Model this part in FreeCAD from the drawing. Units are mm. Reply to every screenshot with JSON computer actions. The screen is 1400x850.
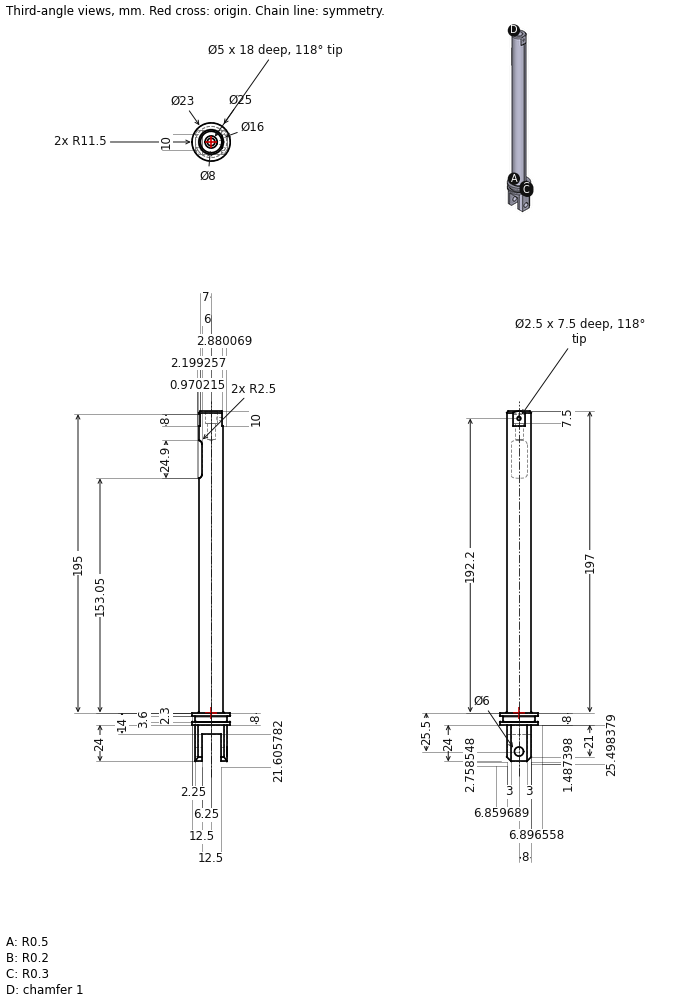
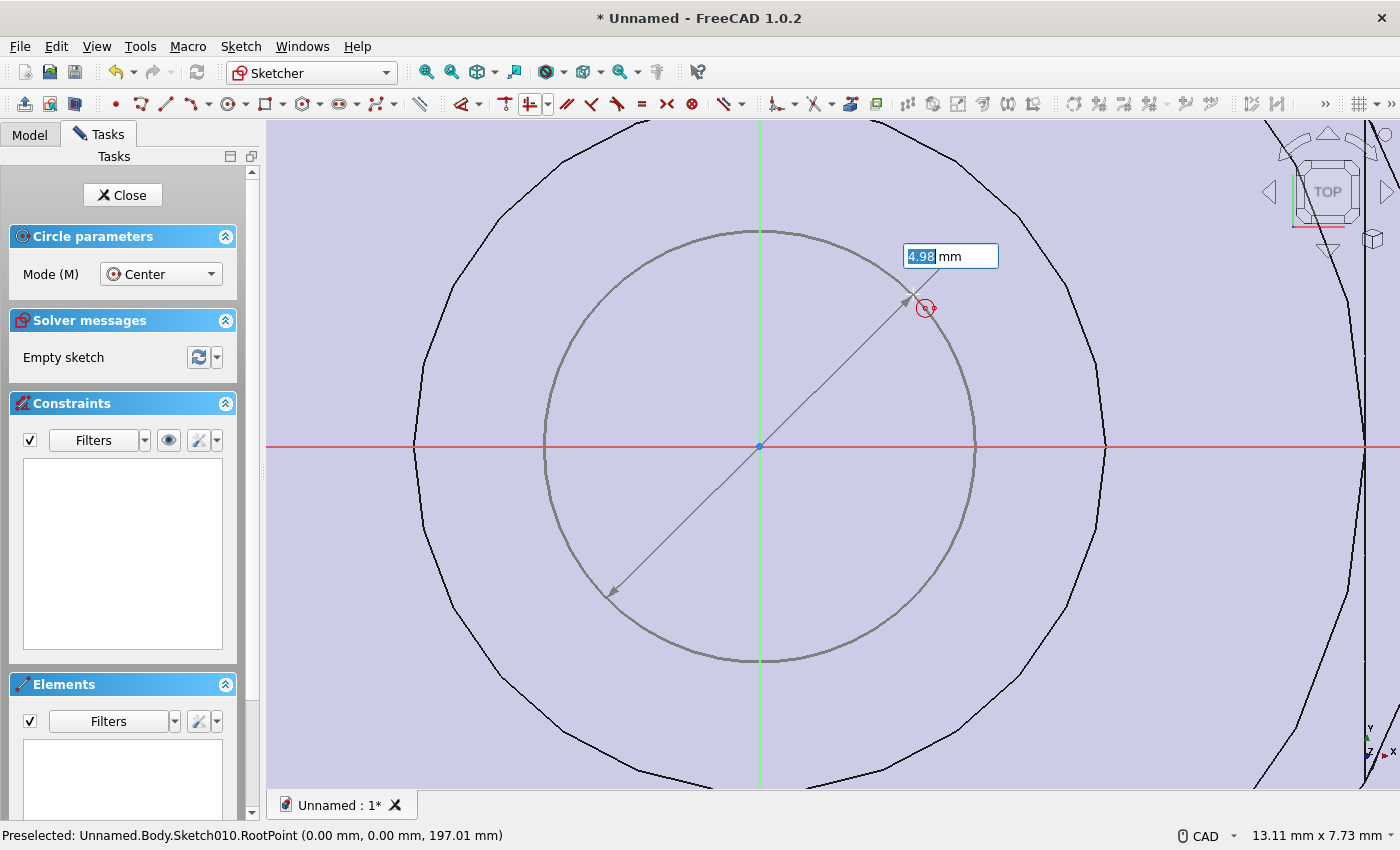
{"action": "type", "text": "5"}
{"action": "key", "text": "Return"}
{"action": "key", "text": "Escape"}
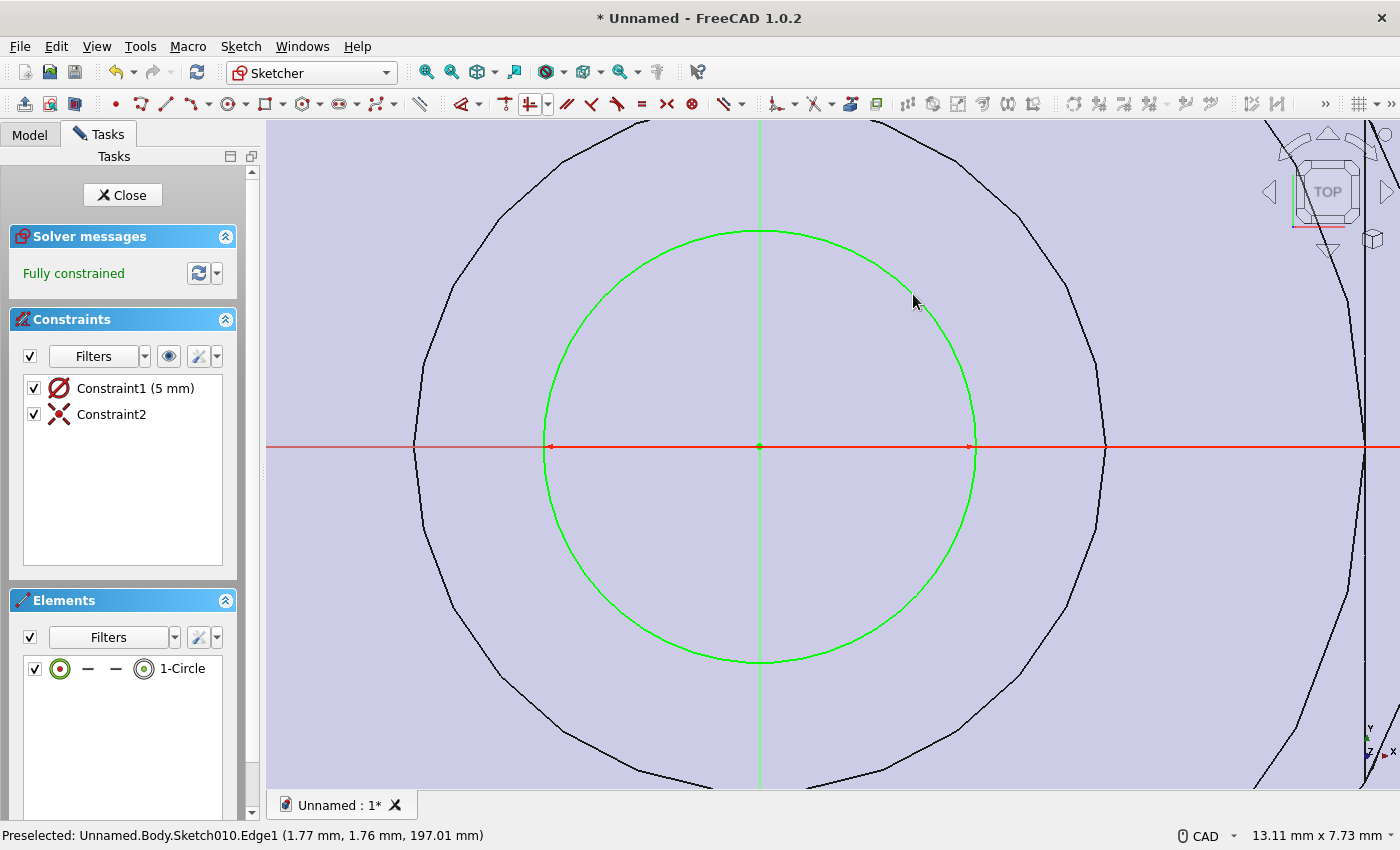
{"action": "left_click", "coordinate": [123, 195]}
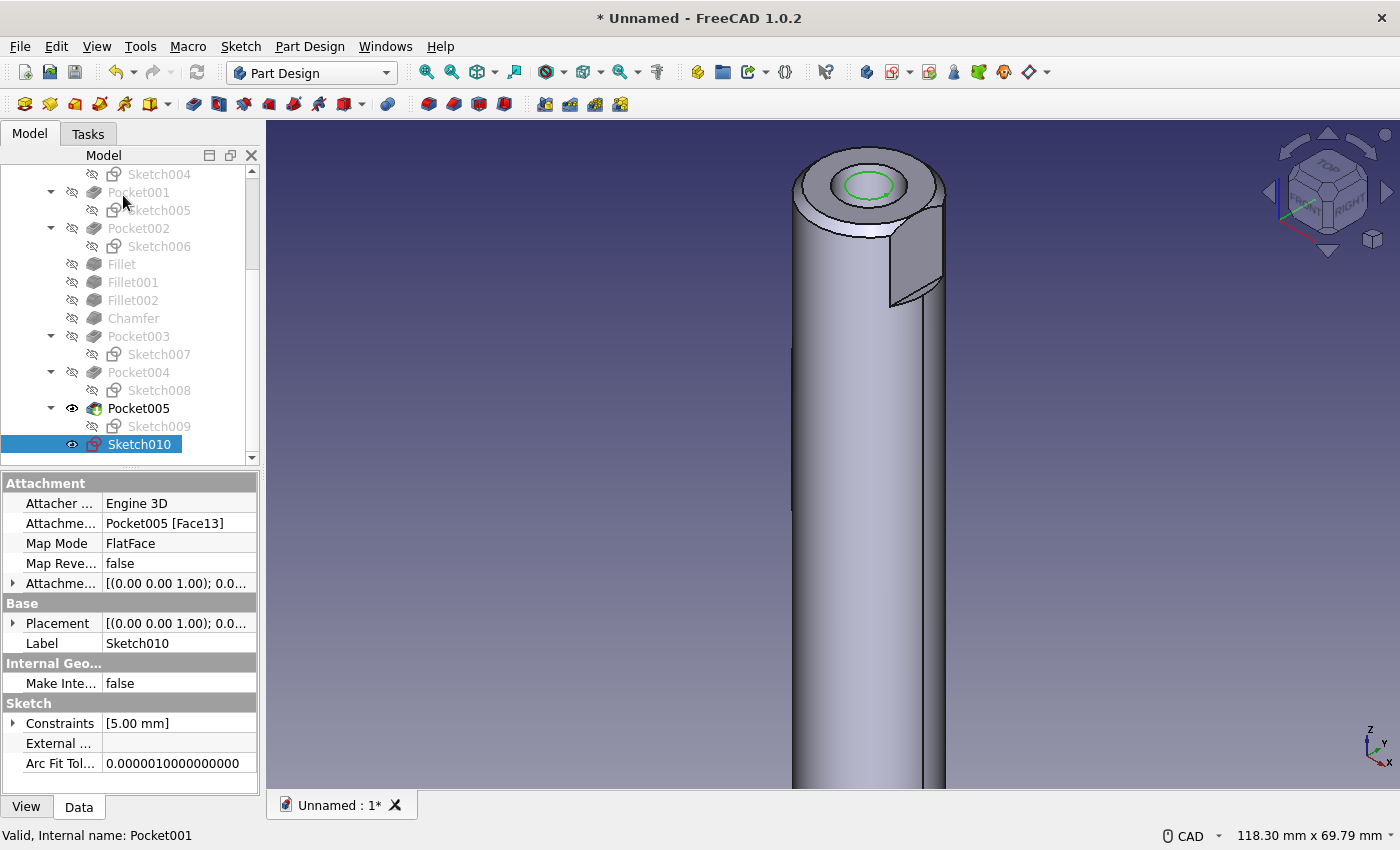
{"action": "left_click", "coordinate": [219, 104]}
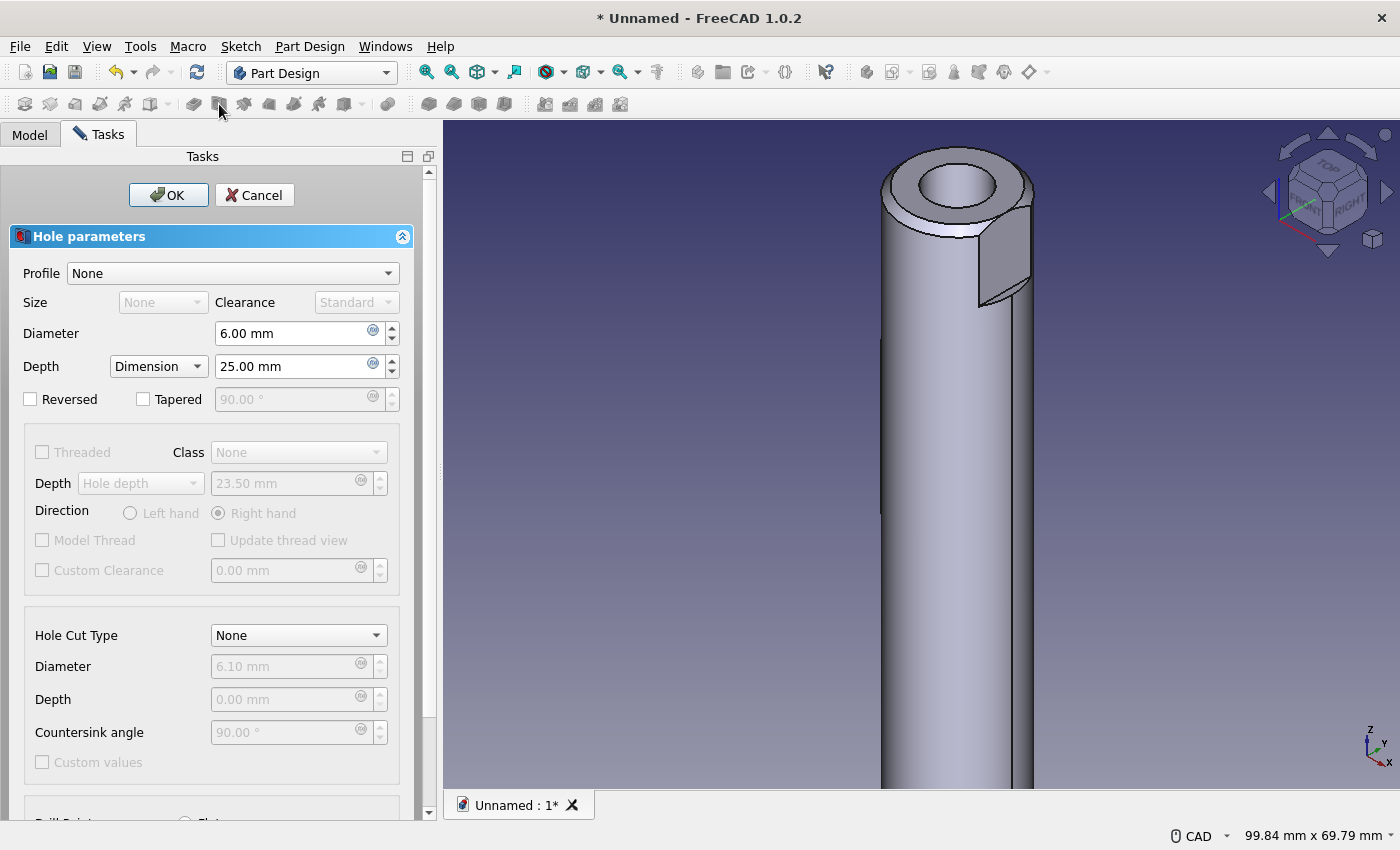
{"action": "triple_click", "coordinate": [300, 334]}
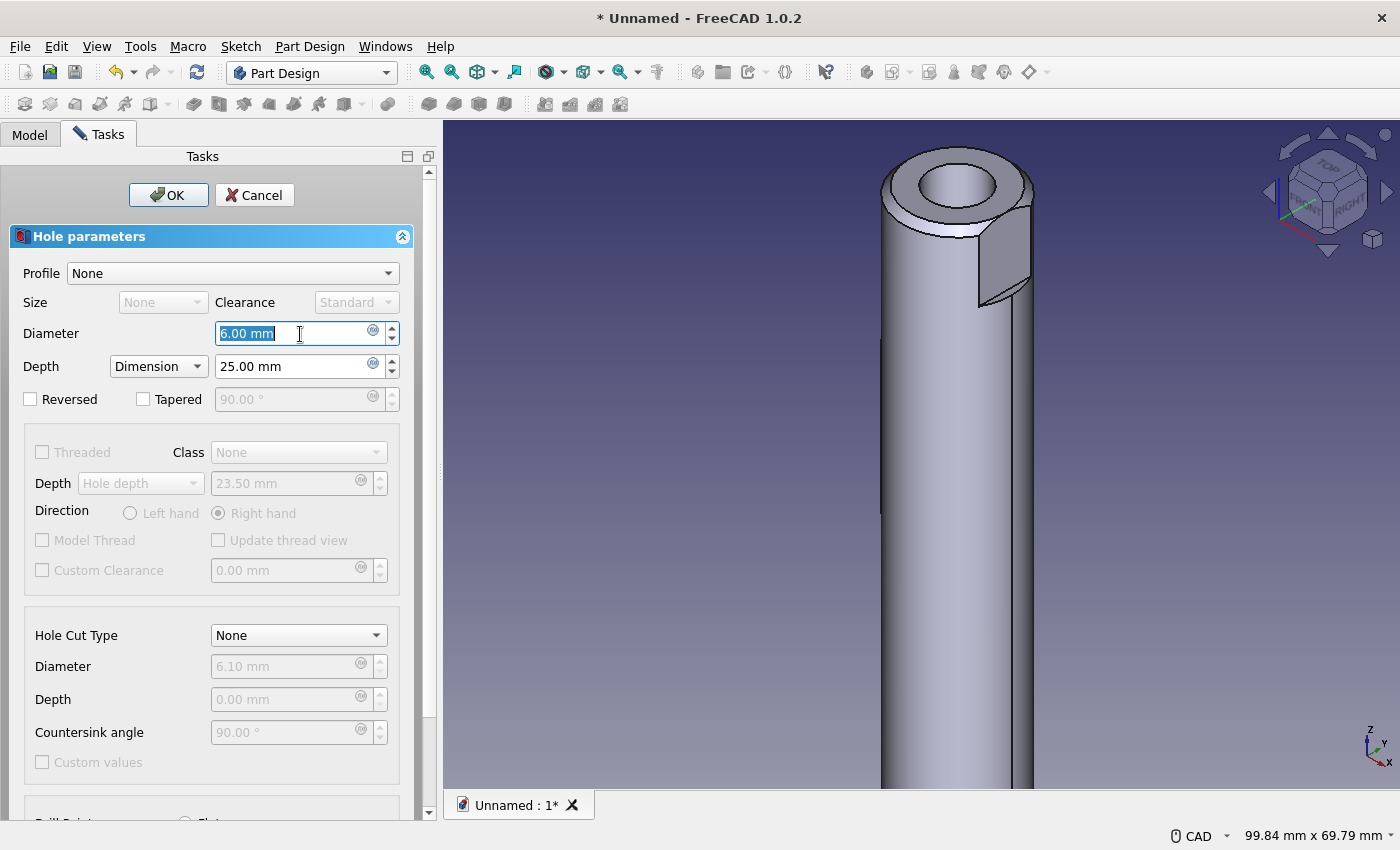
{"action": "type", "text": "5"}
{"action": "key", "text": "Tab"}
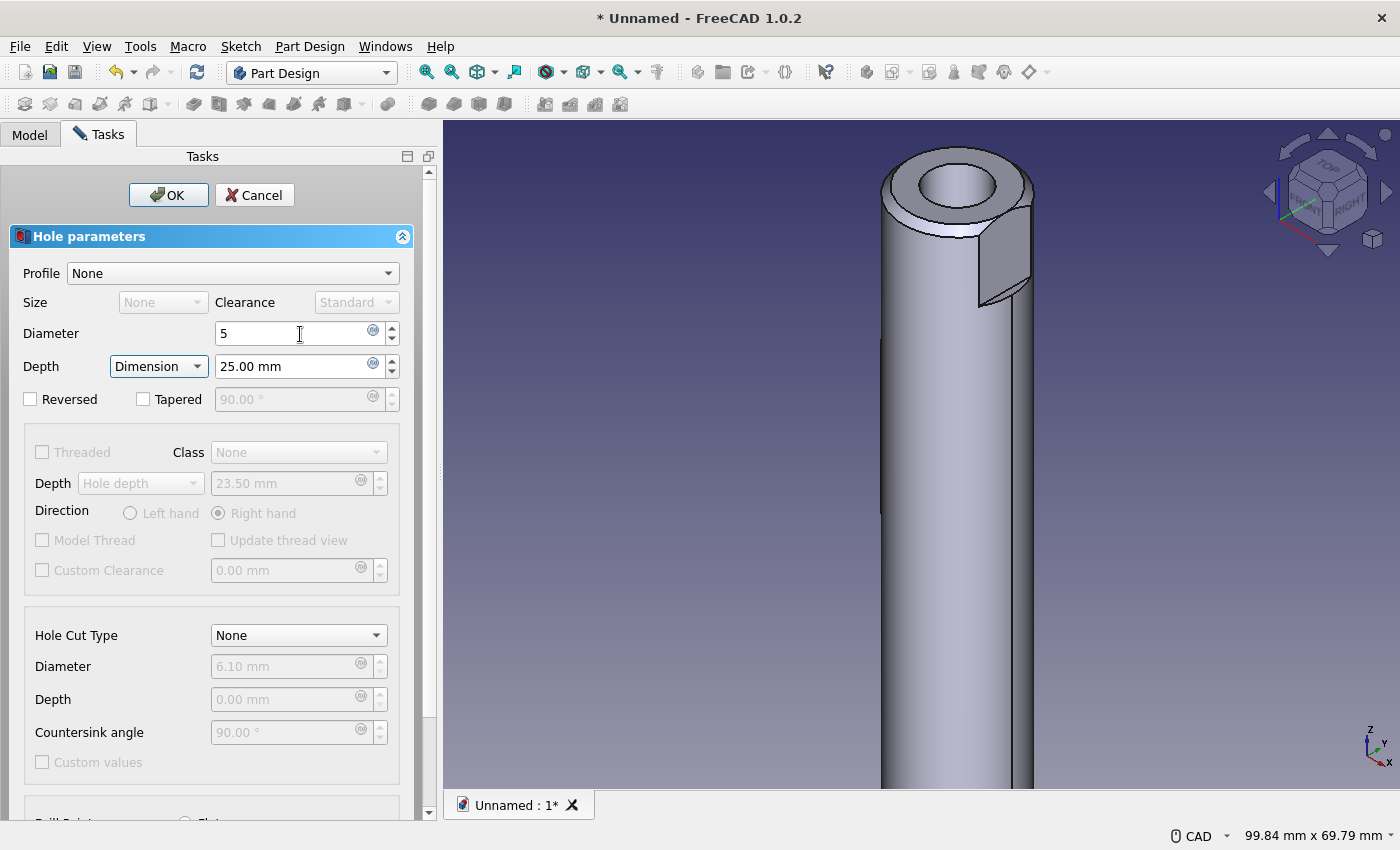
{"action": "triple_click", "coordinate": [300, 366]}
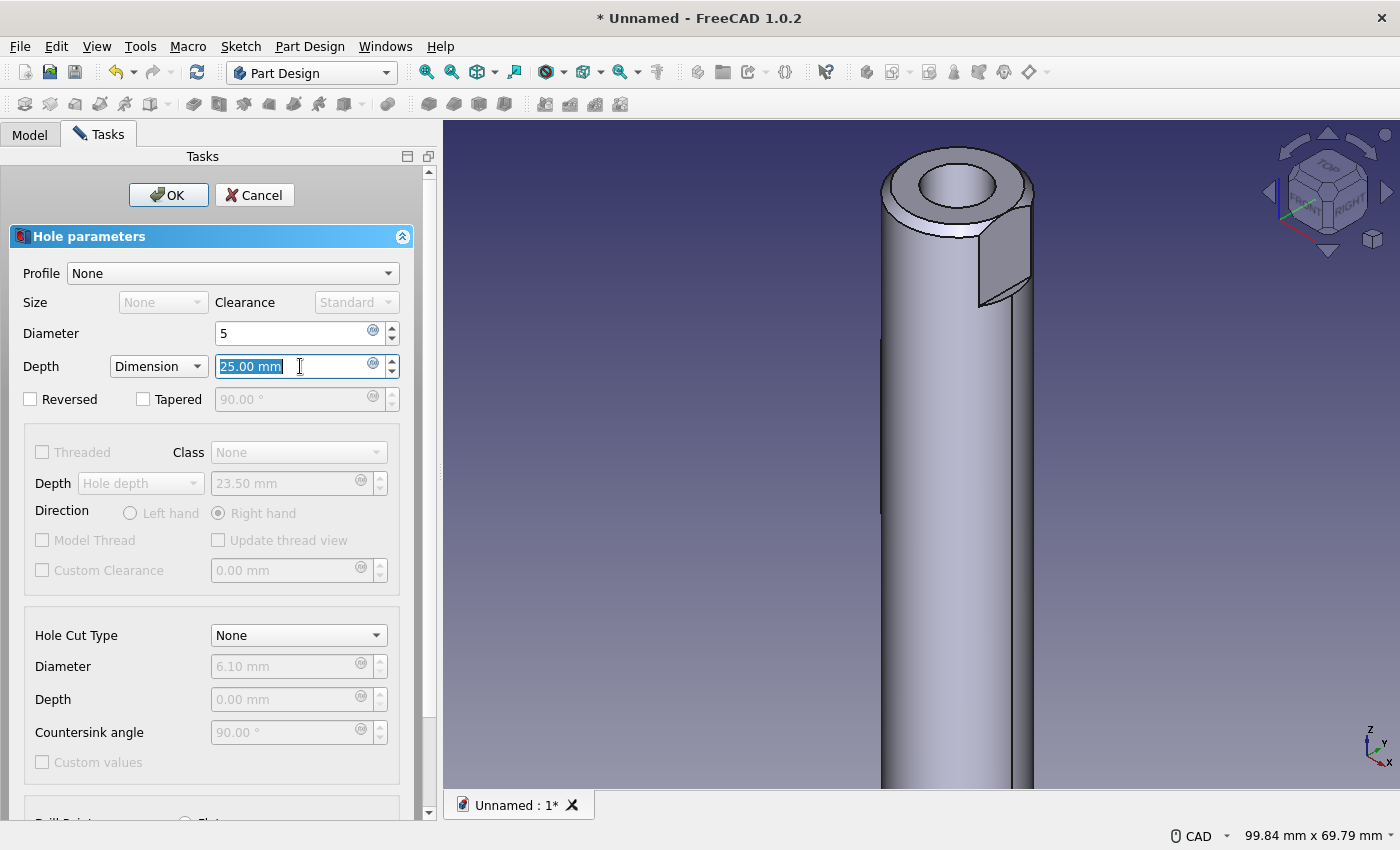
{"action": "type", "text": "18"}
{"action": "key", "text": "Tab"}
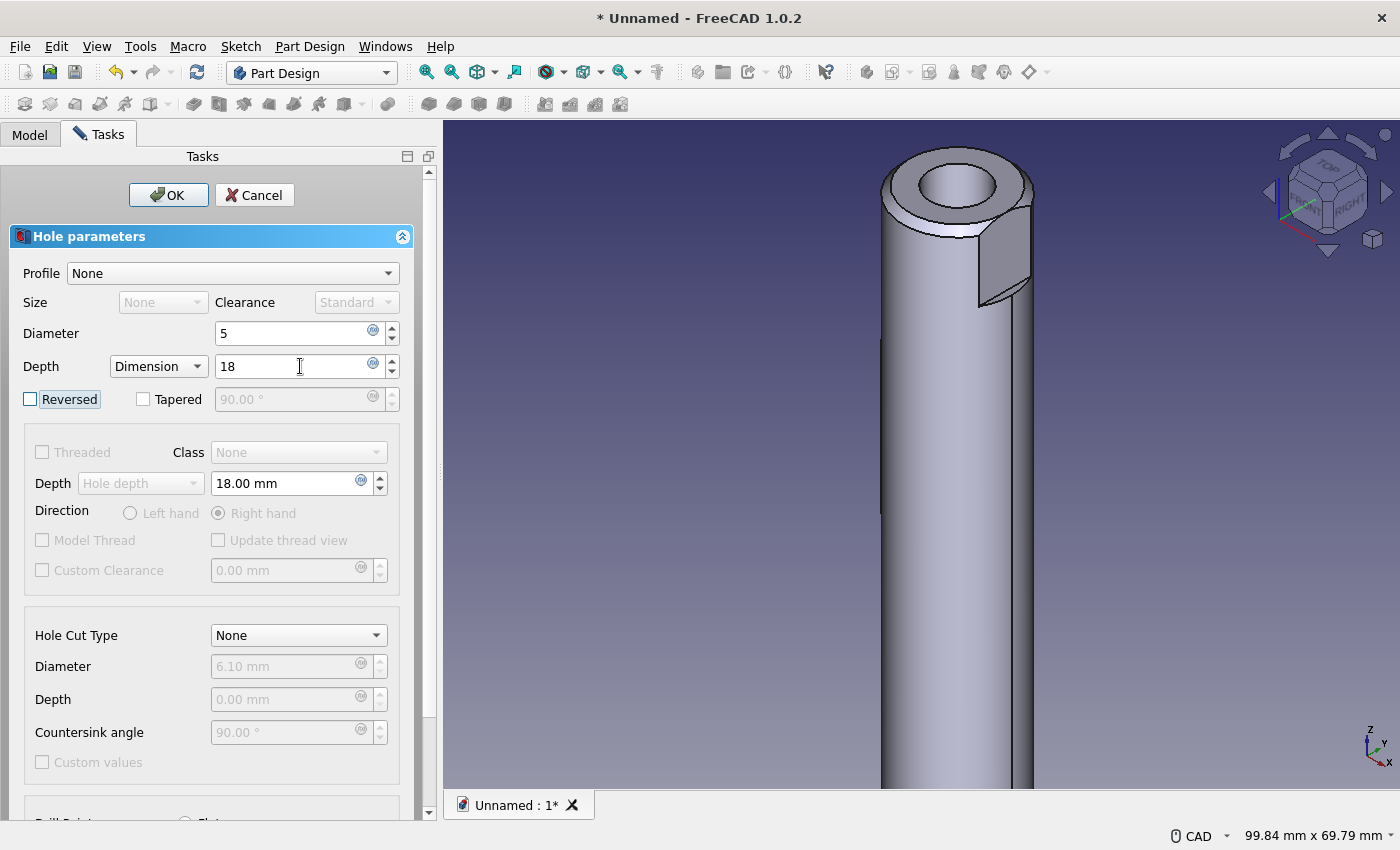
{"action": "left_click", "coordinate": [169, 195]}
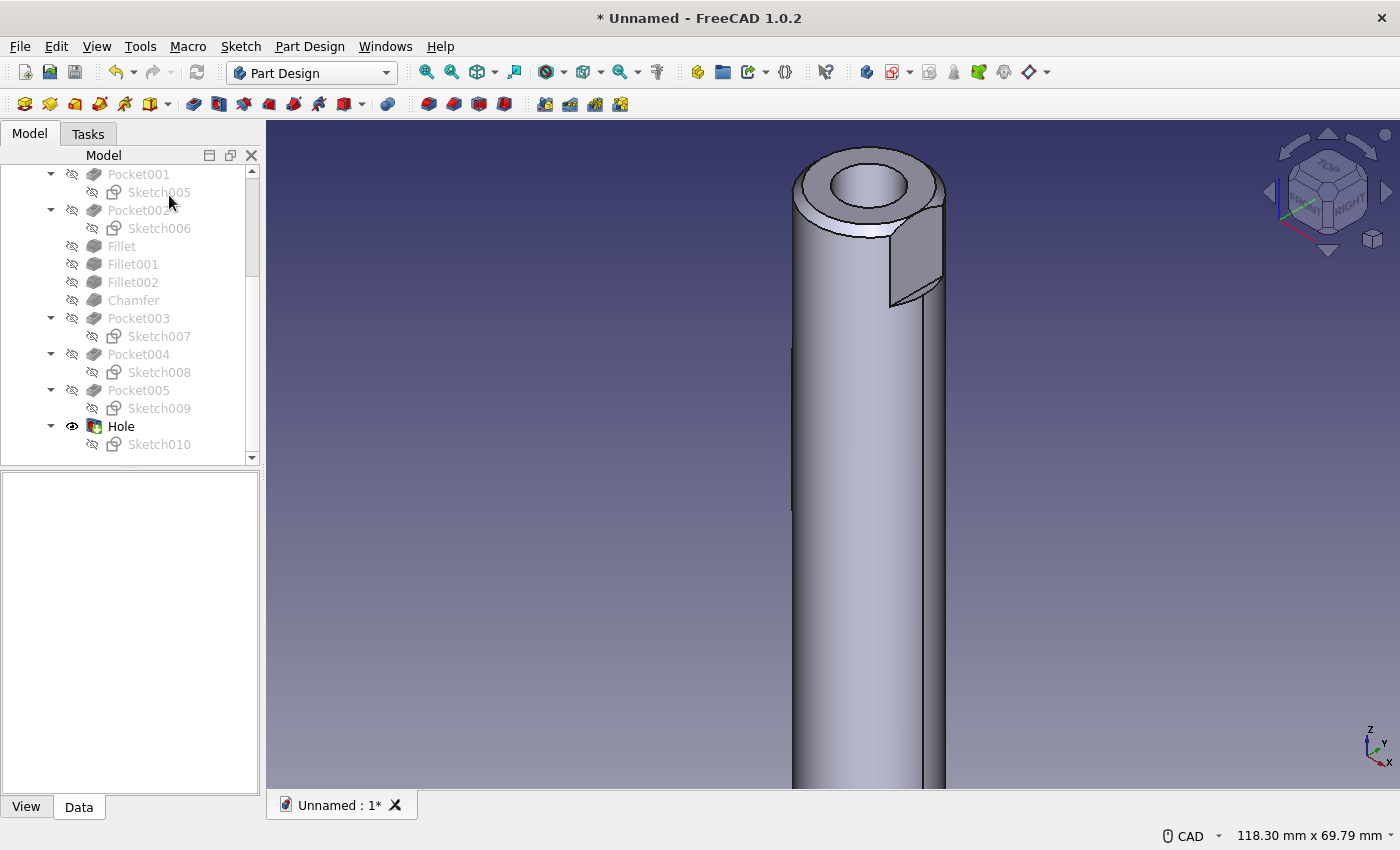
{"action": "left_click", "coordinate": [427, 72]}